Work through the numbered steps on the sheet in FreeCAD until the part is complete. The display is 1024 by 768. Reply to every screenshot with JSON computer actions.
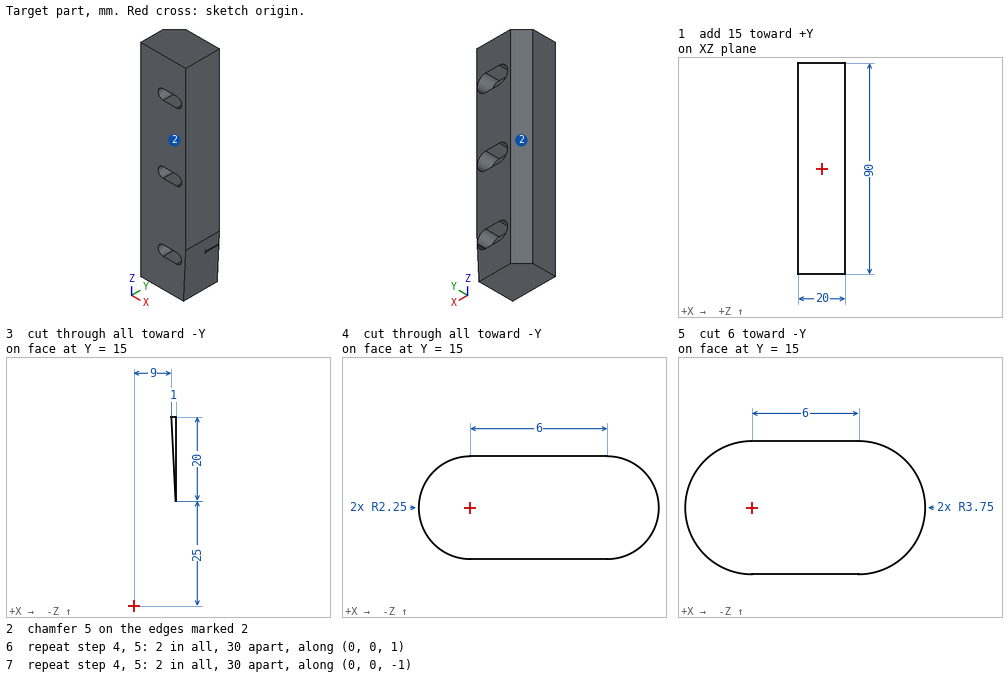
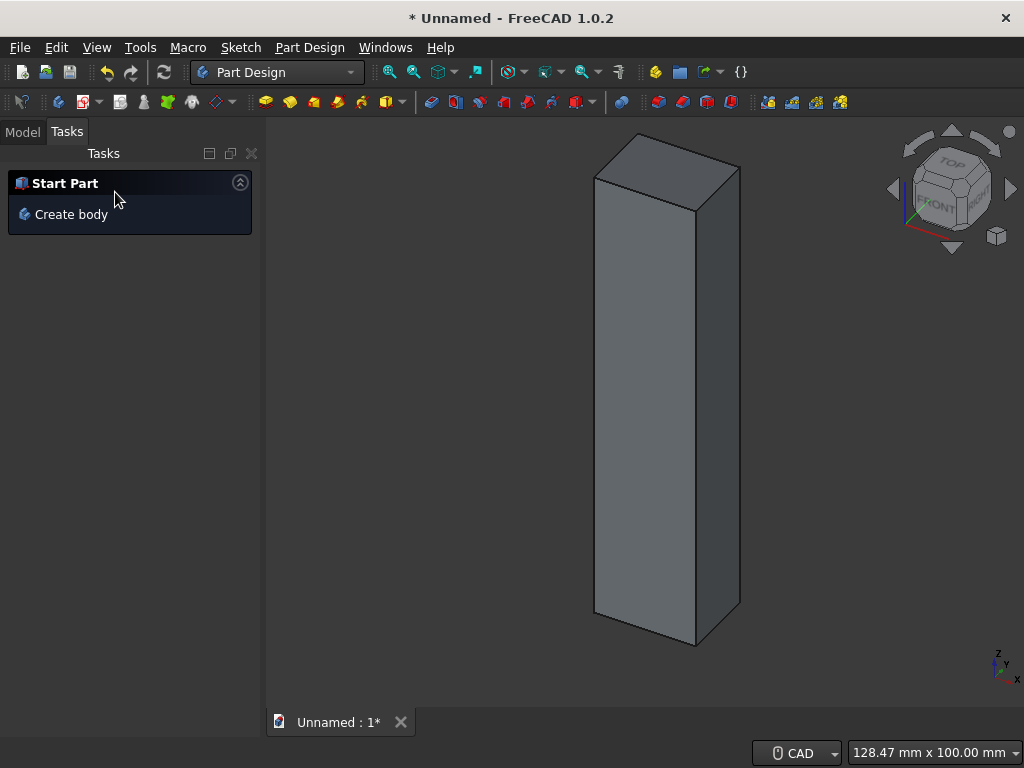
{"action": "key", "text": "0"}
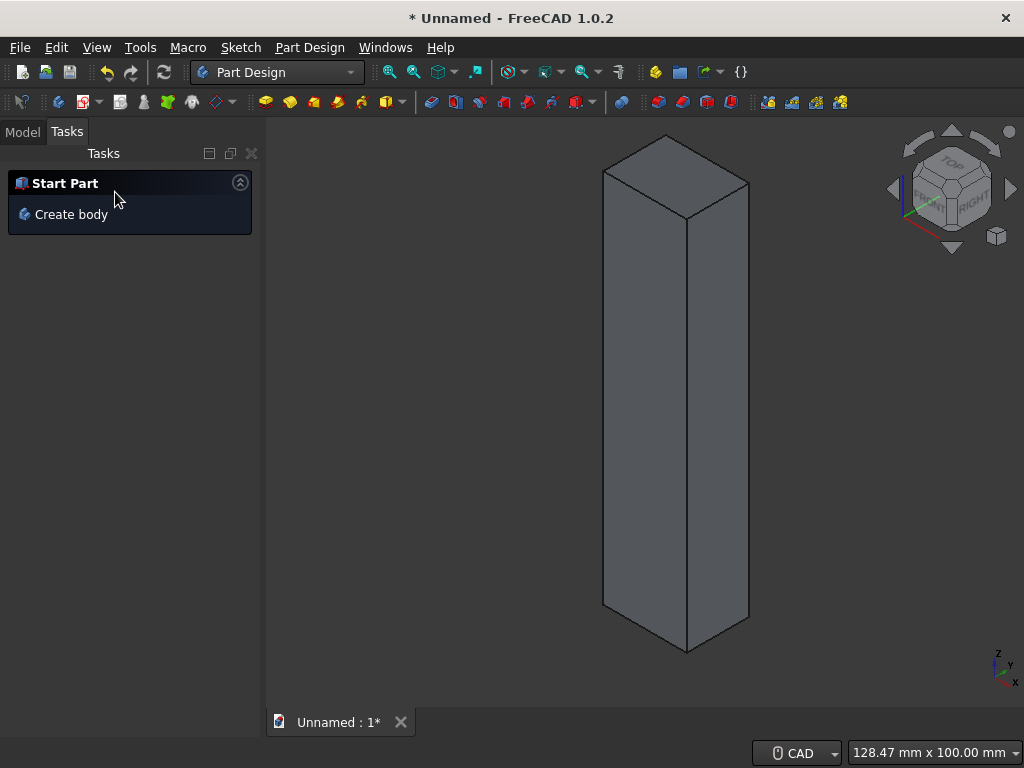
{"action": "key", "text": "2"}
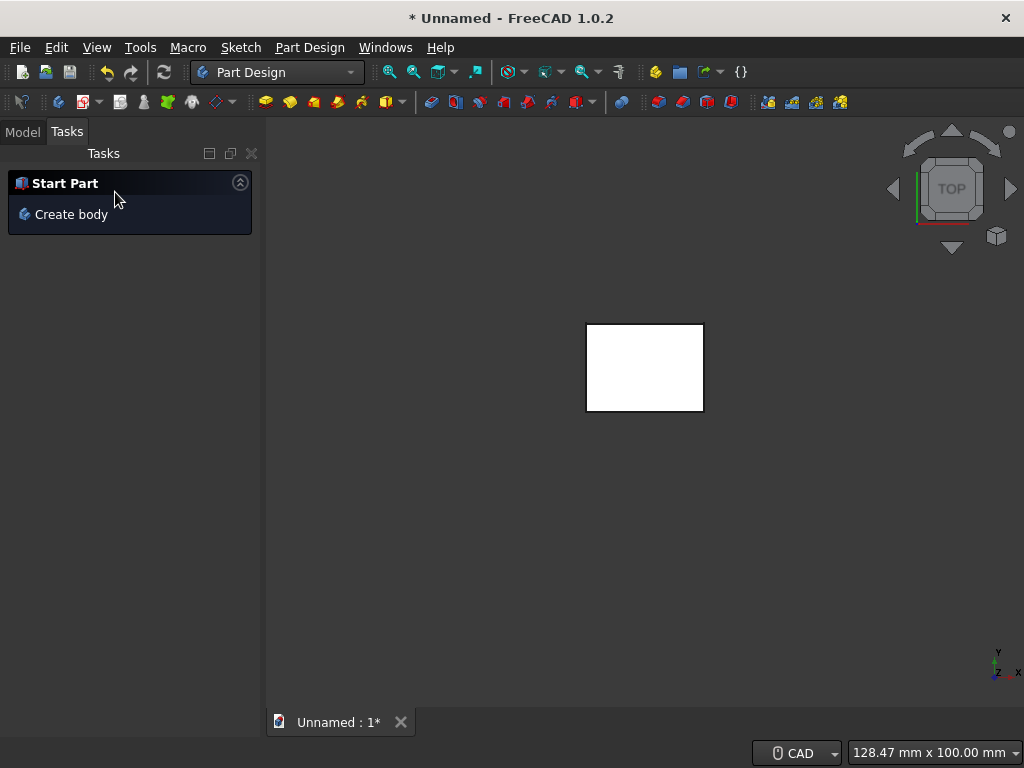
{"action": "left_click", "coordinate": [390, 72]}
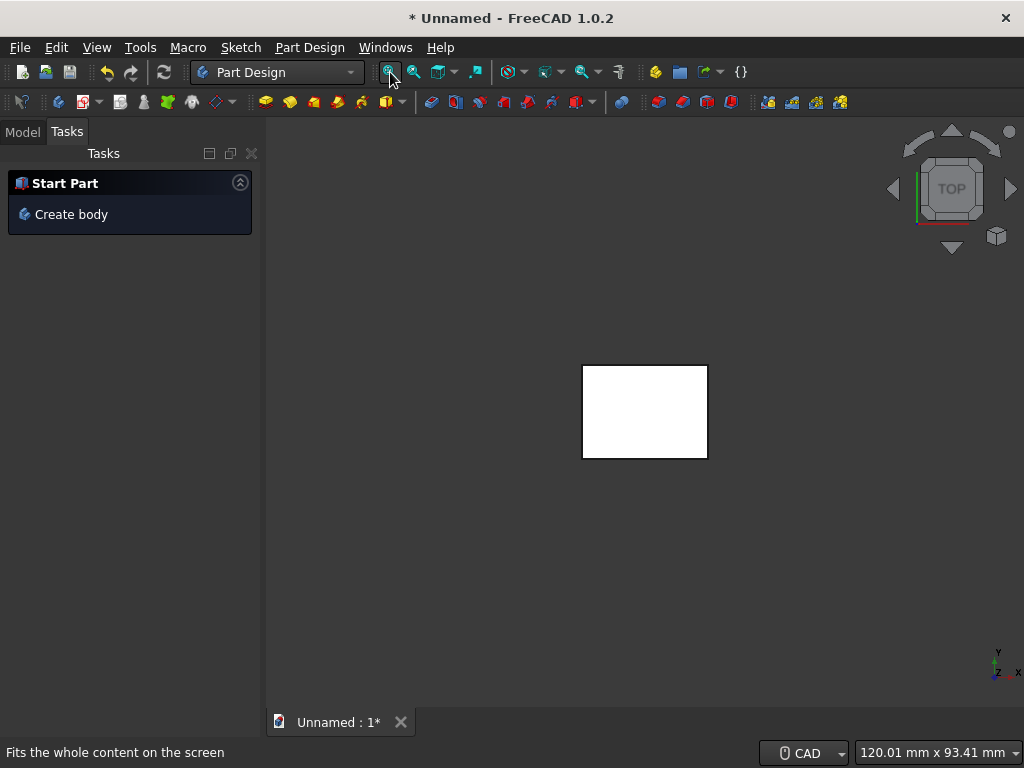
{"action": "key", "text": "1"}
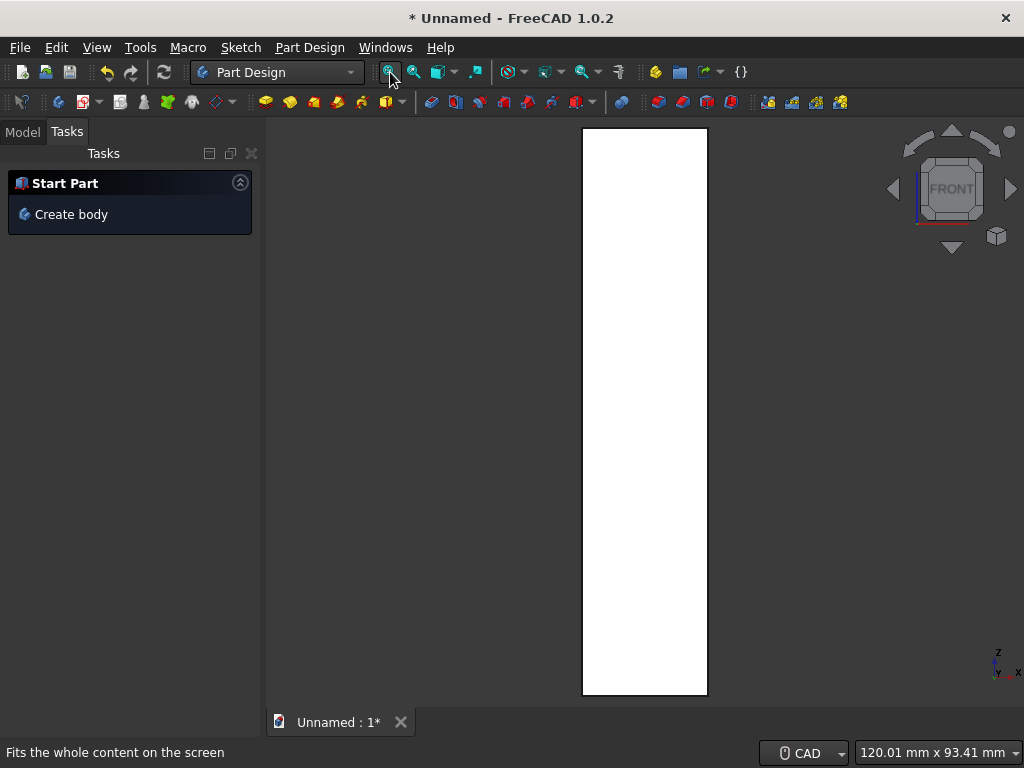
{"action": "key", "text": "3"}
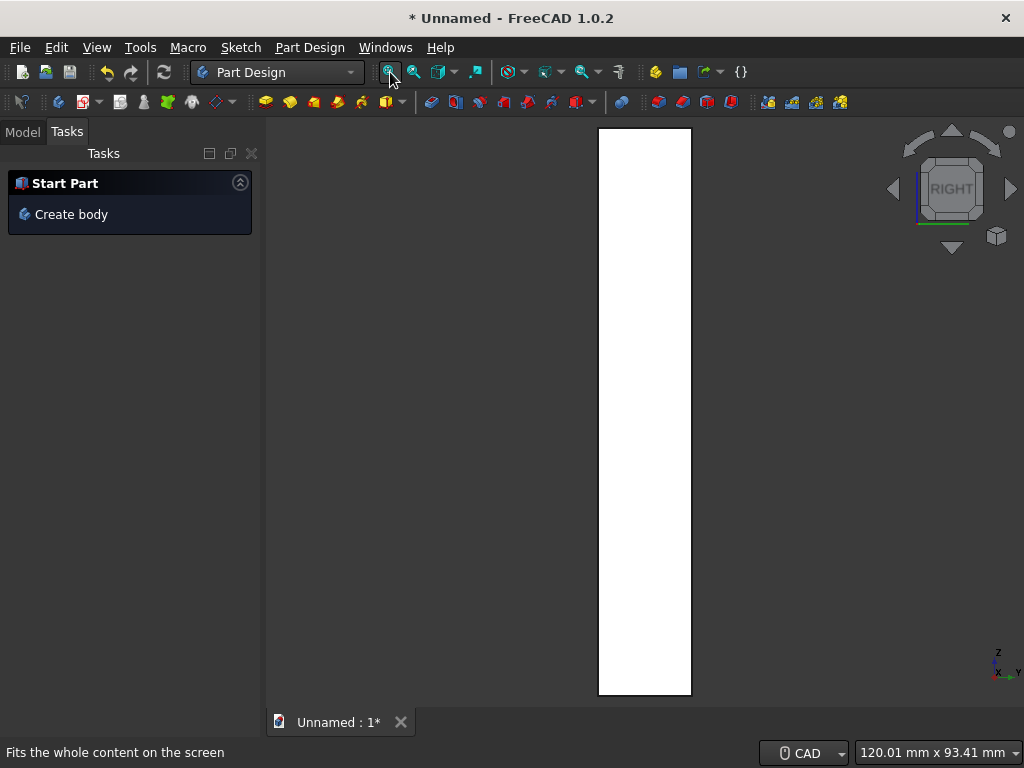
{"action": "key", "text": "5"}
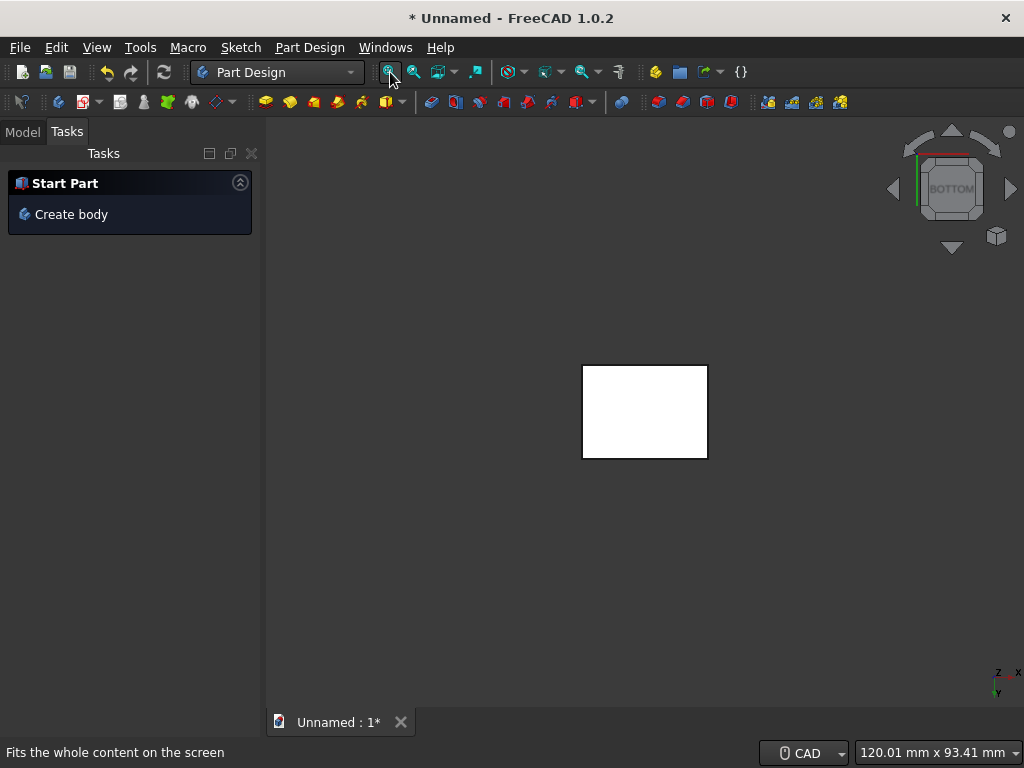
{"action": "left_click", "coordinate": [390, 72]}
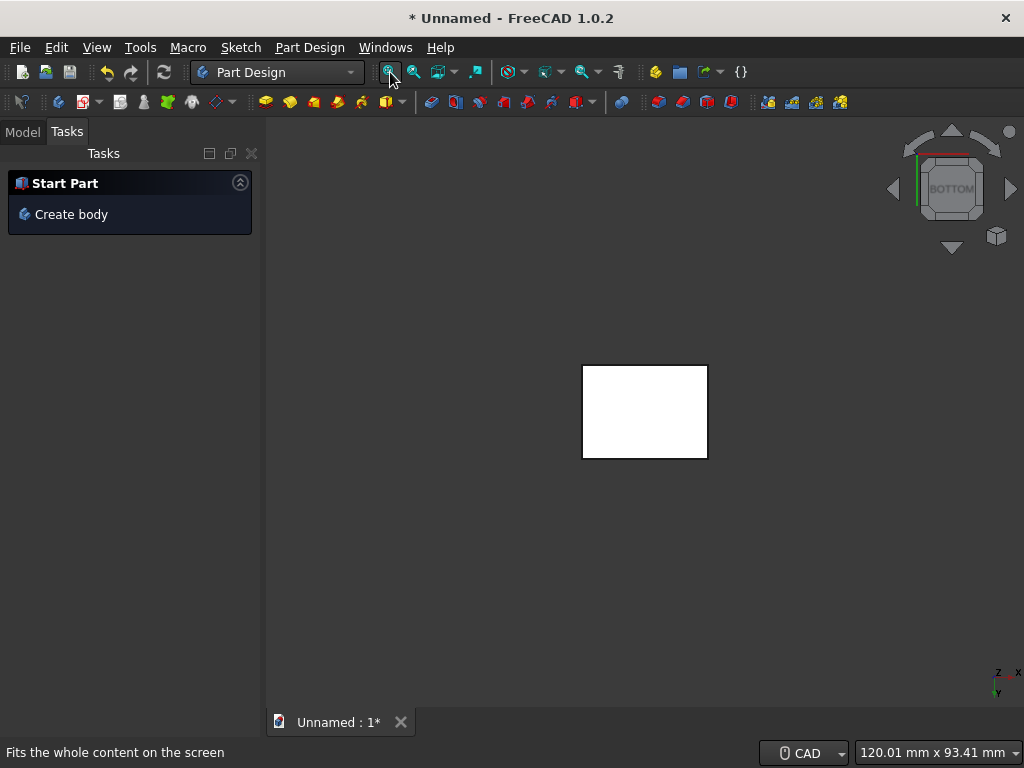
{"action": "key", "text": "4"}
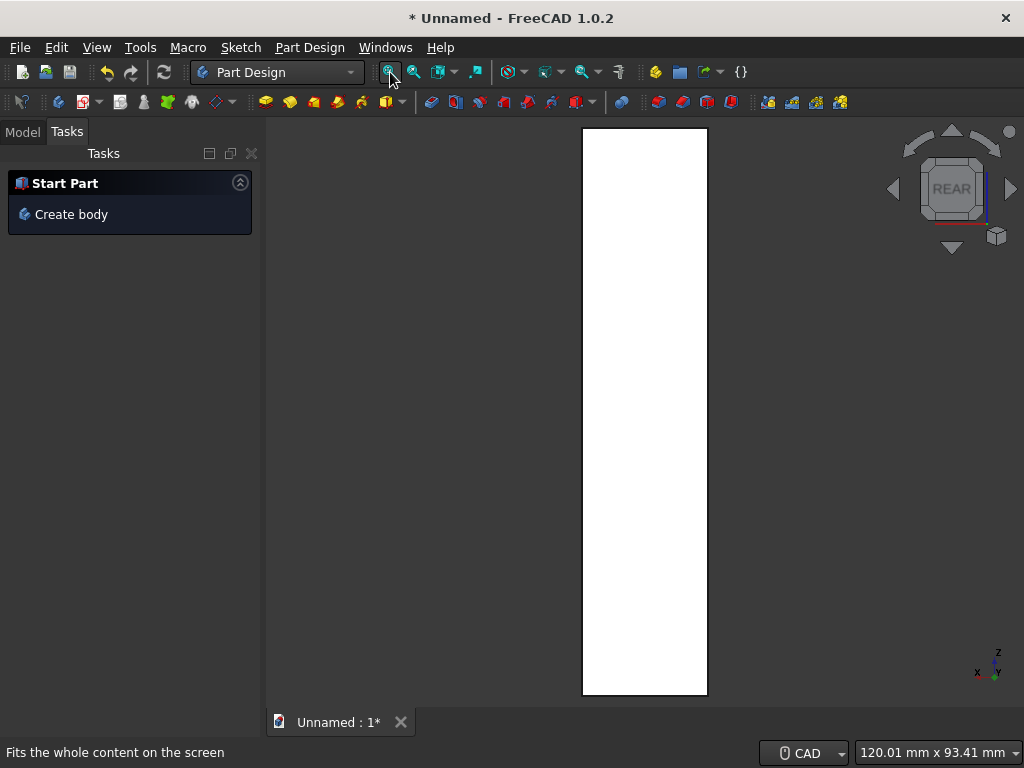
{"action": "left_click", "coordinate": [708, 411]}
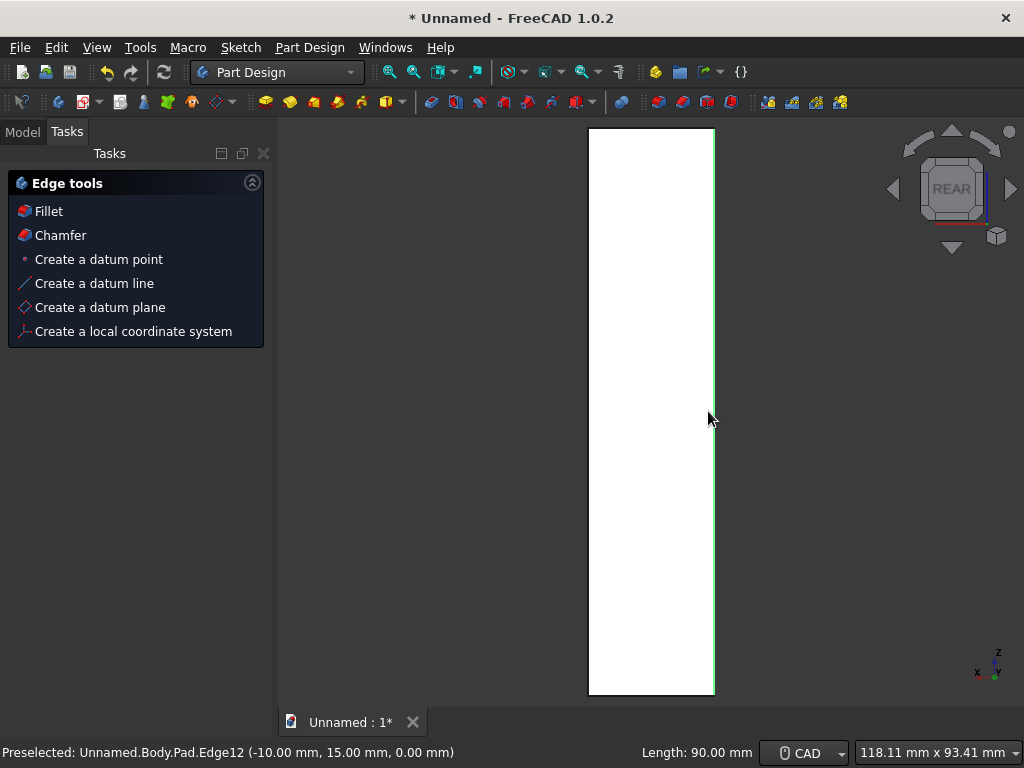
{"action": "left_click", "coordinate": [684, 102]}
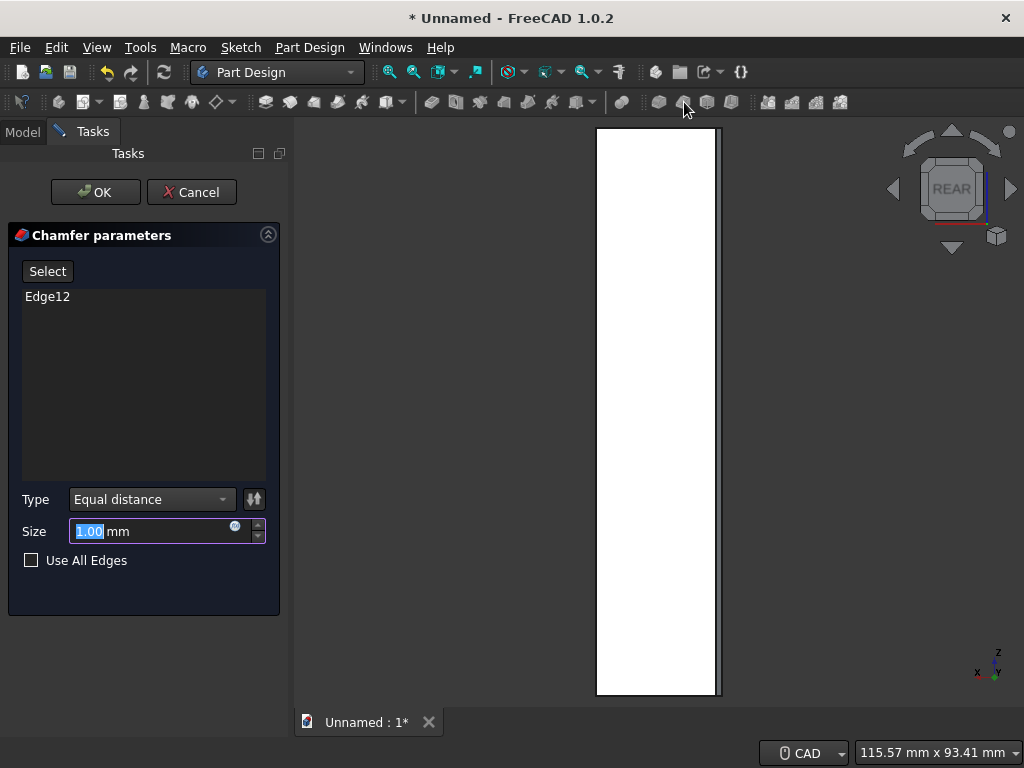
{"action": "type", "text": "5"}
{"action": "key", "text": "Tab"}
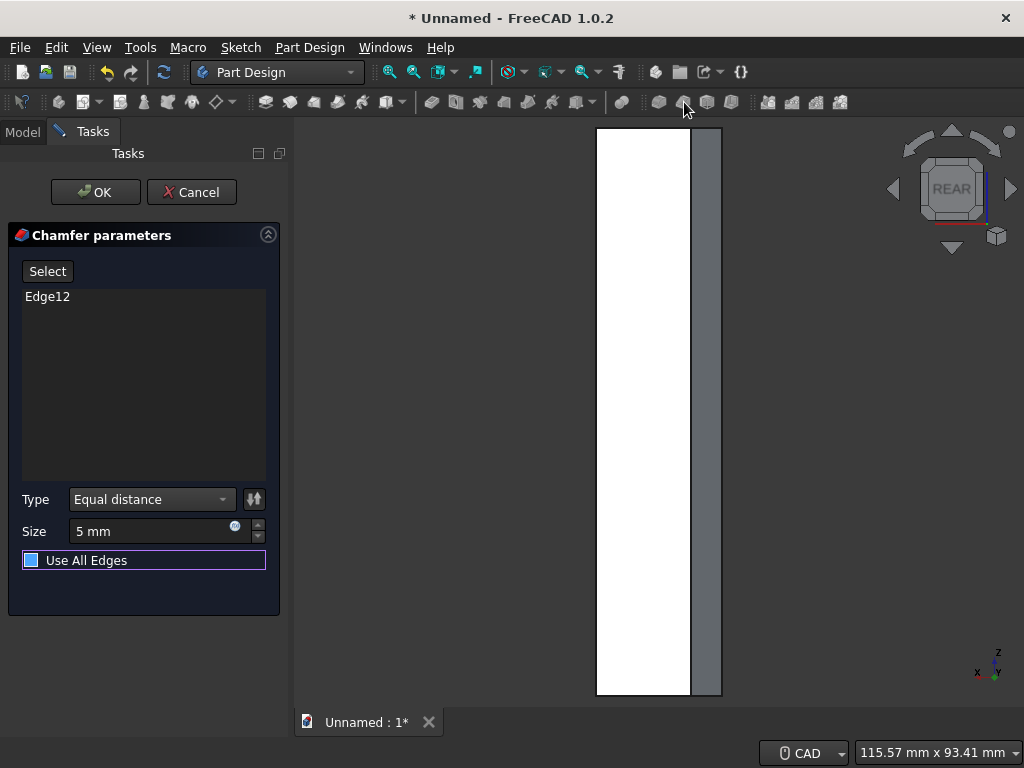
{"action": "left_click", "coordinate": [96, 192]}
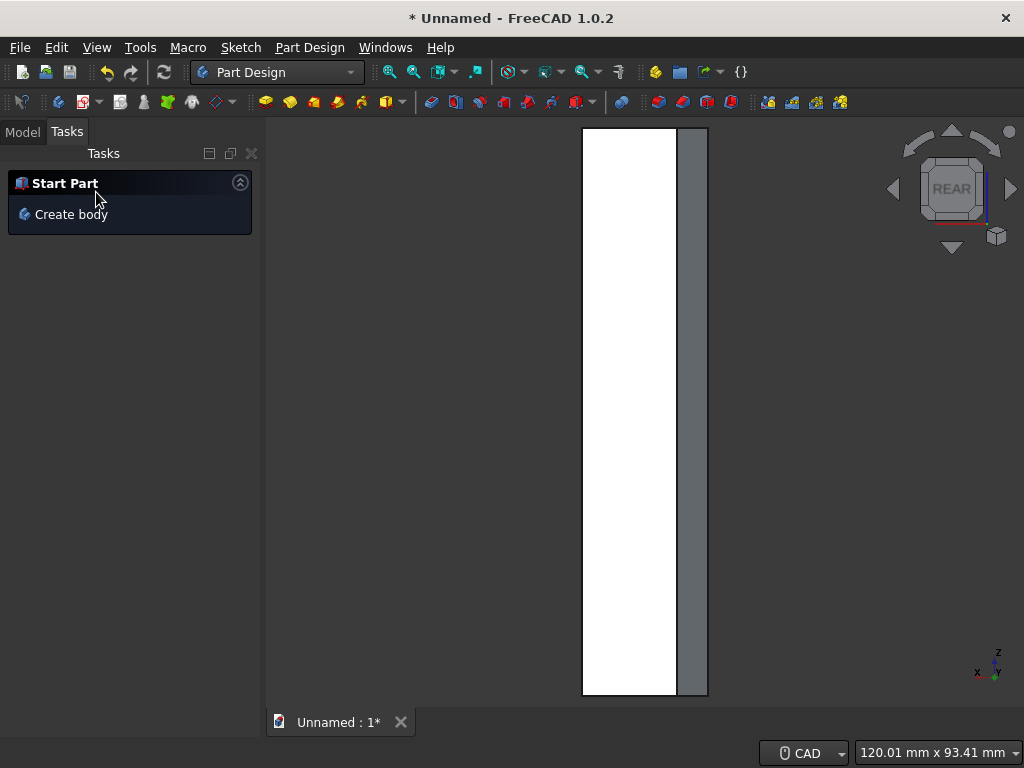
{"action": "left_click", "coordinate": [629, 249]}